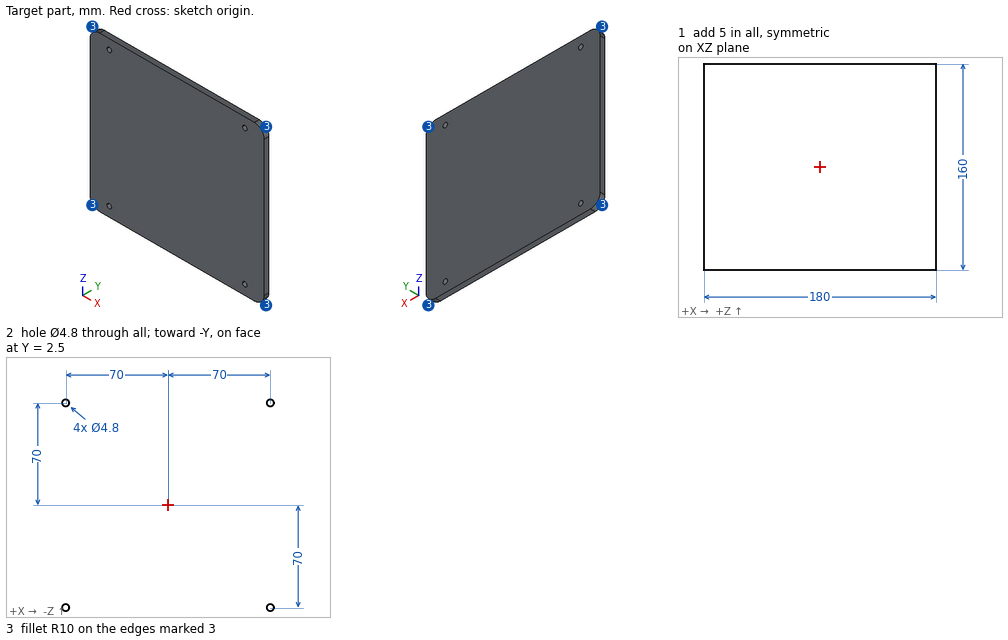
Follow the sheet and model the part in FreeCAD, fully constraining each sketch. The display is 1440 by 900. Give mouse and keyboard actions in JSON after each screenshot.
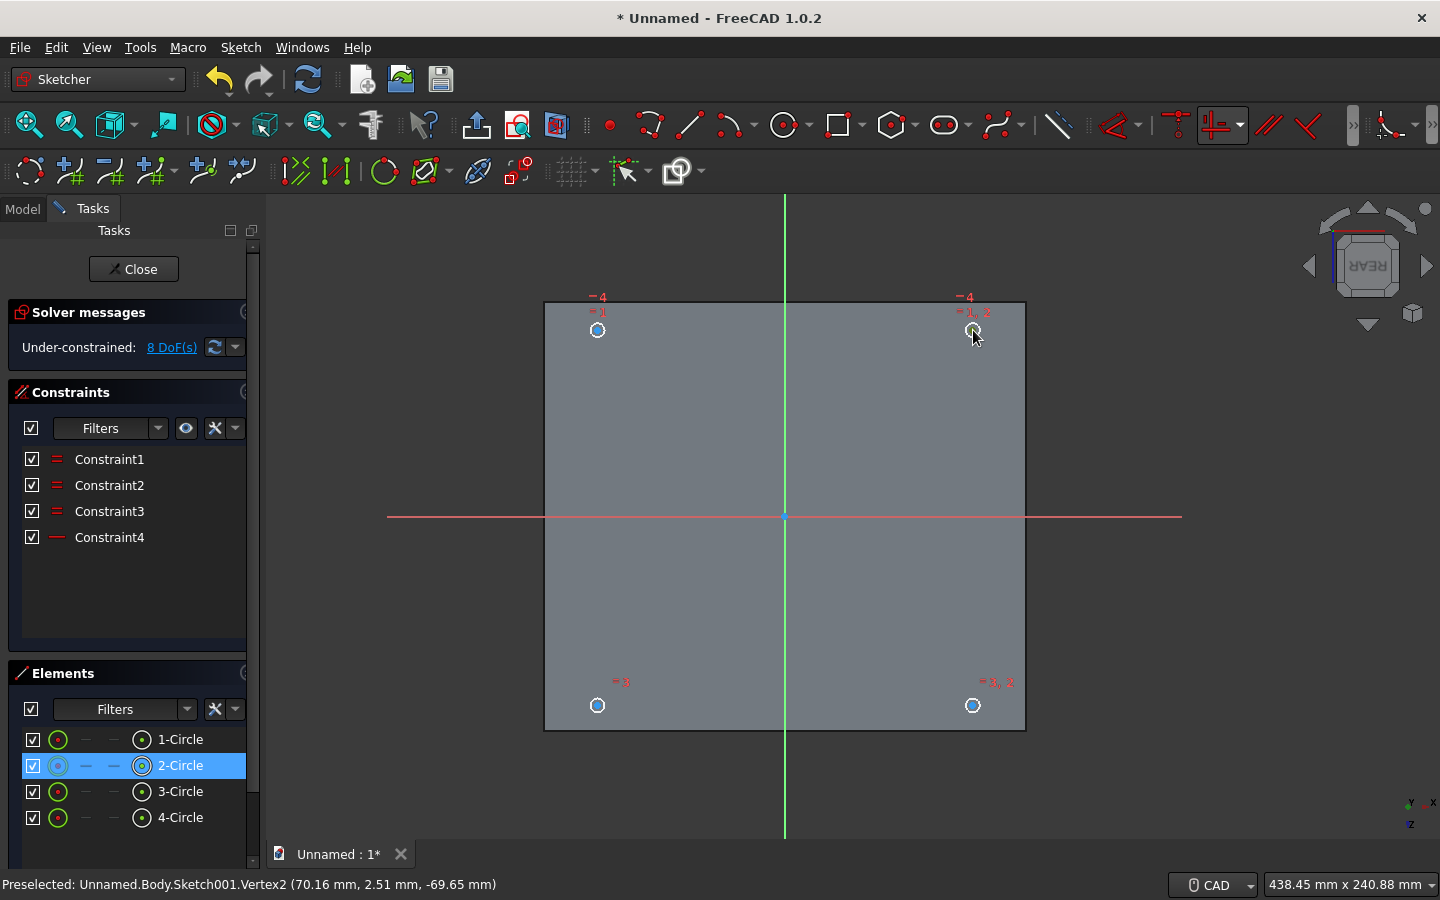
{"action": "left_click", "coordinate": [973, 705]}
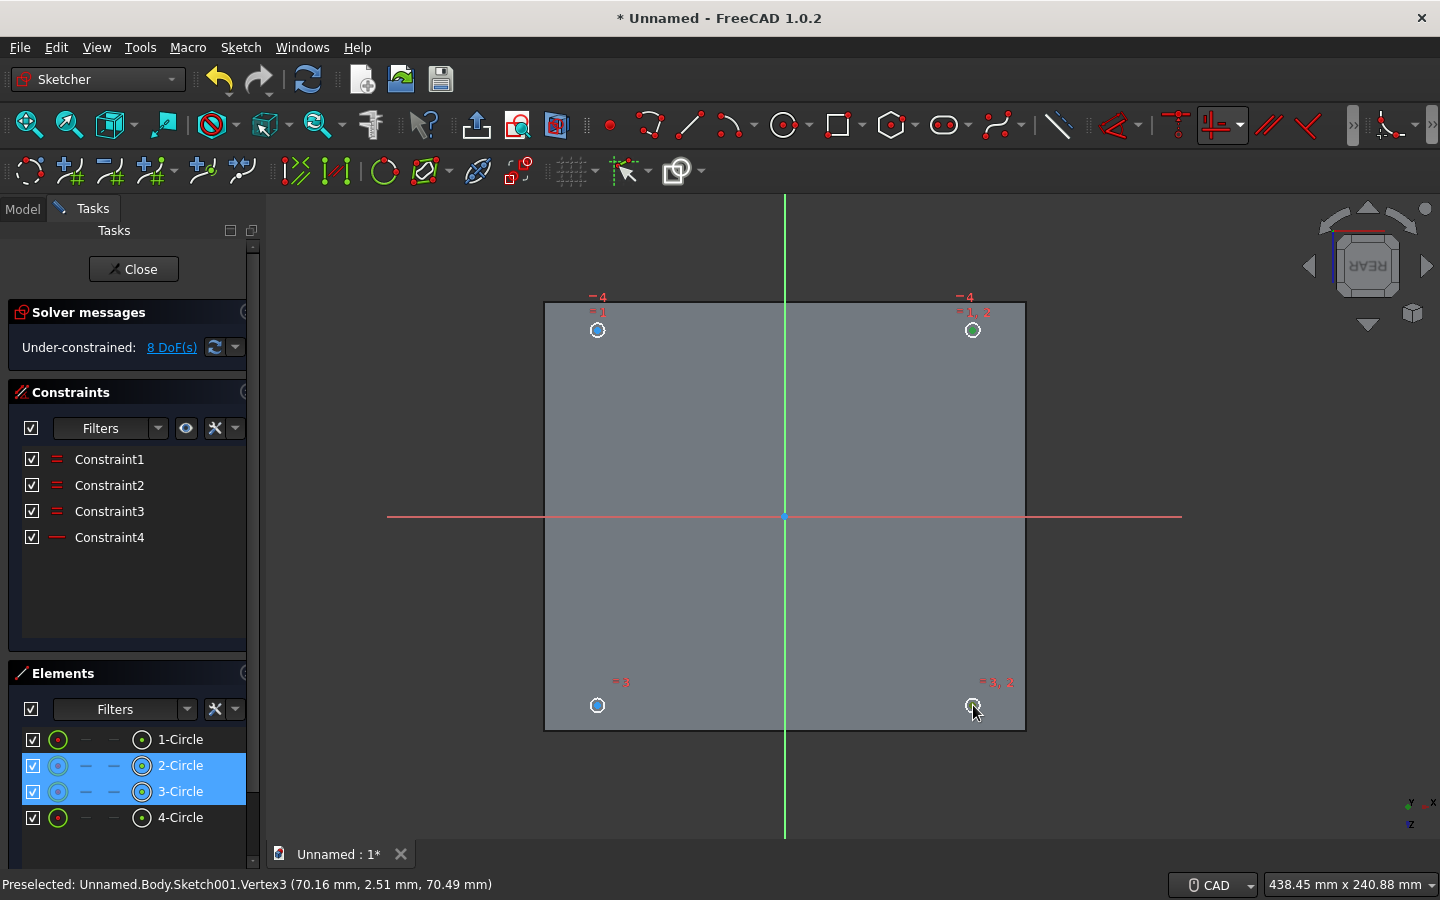
{"action": "key", "text": "v"}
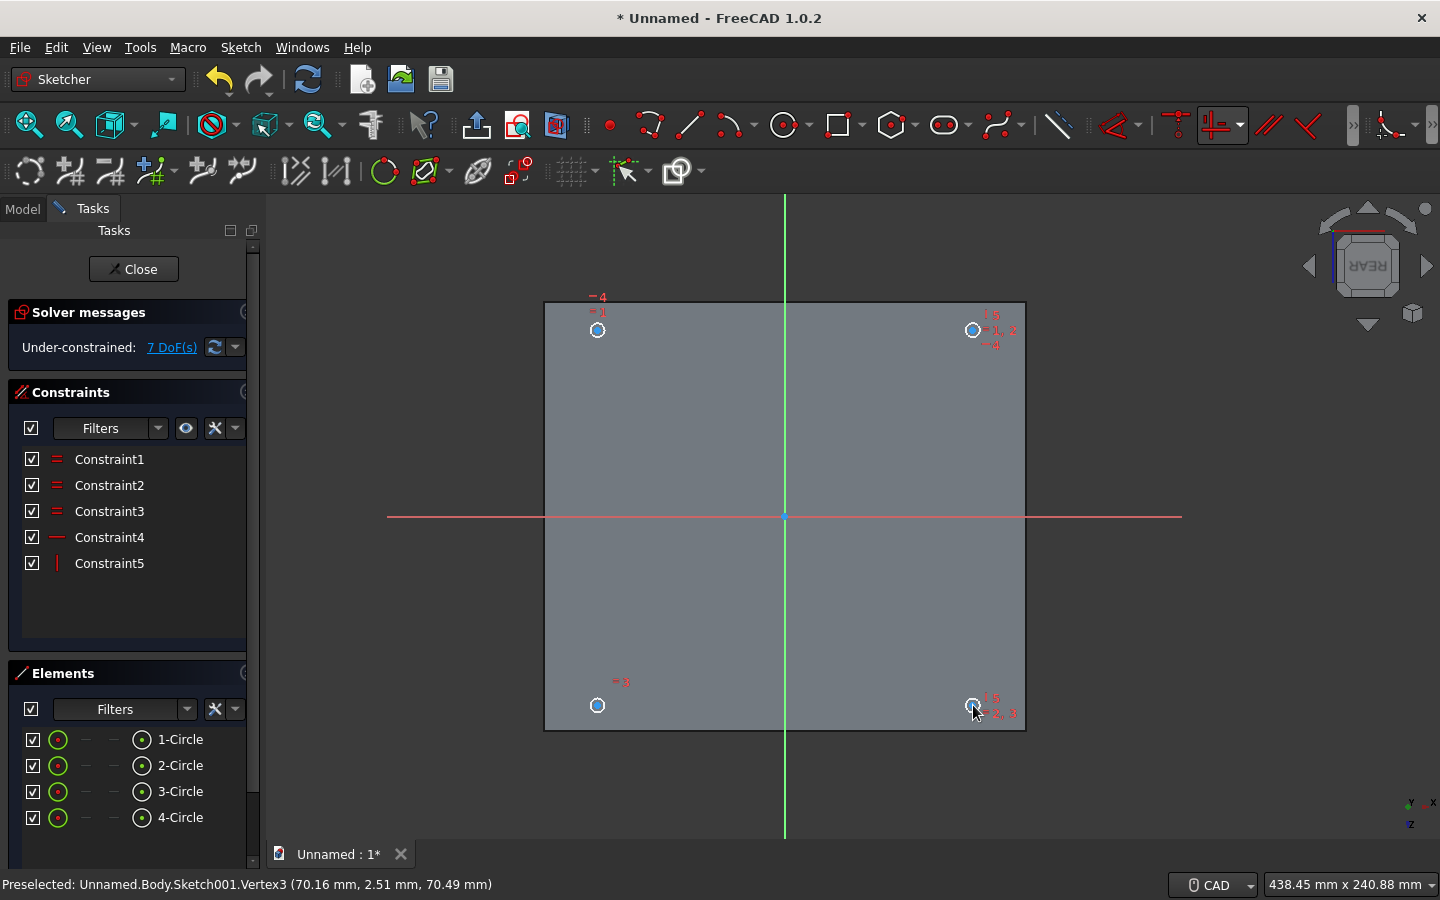
{"action": "left_click", "coordinate": [598, 330]}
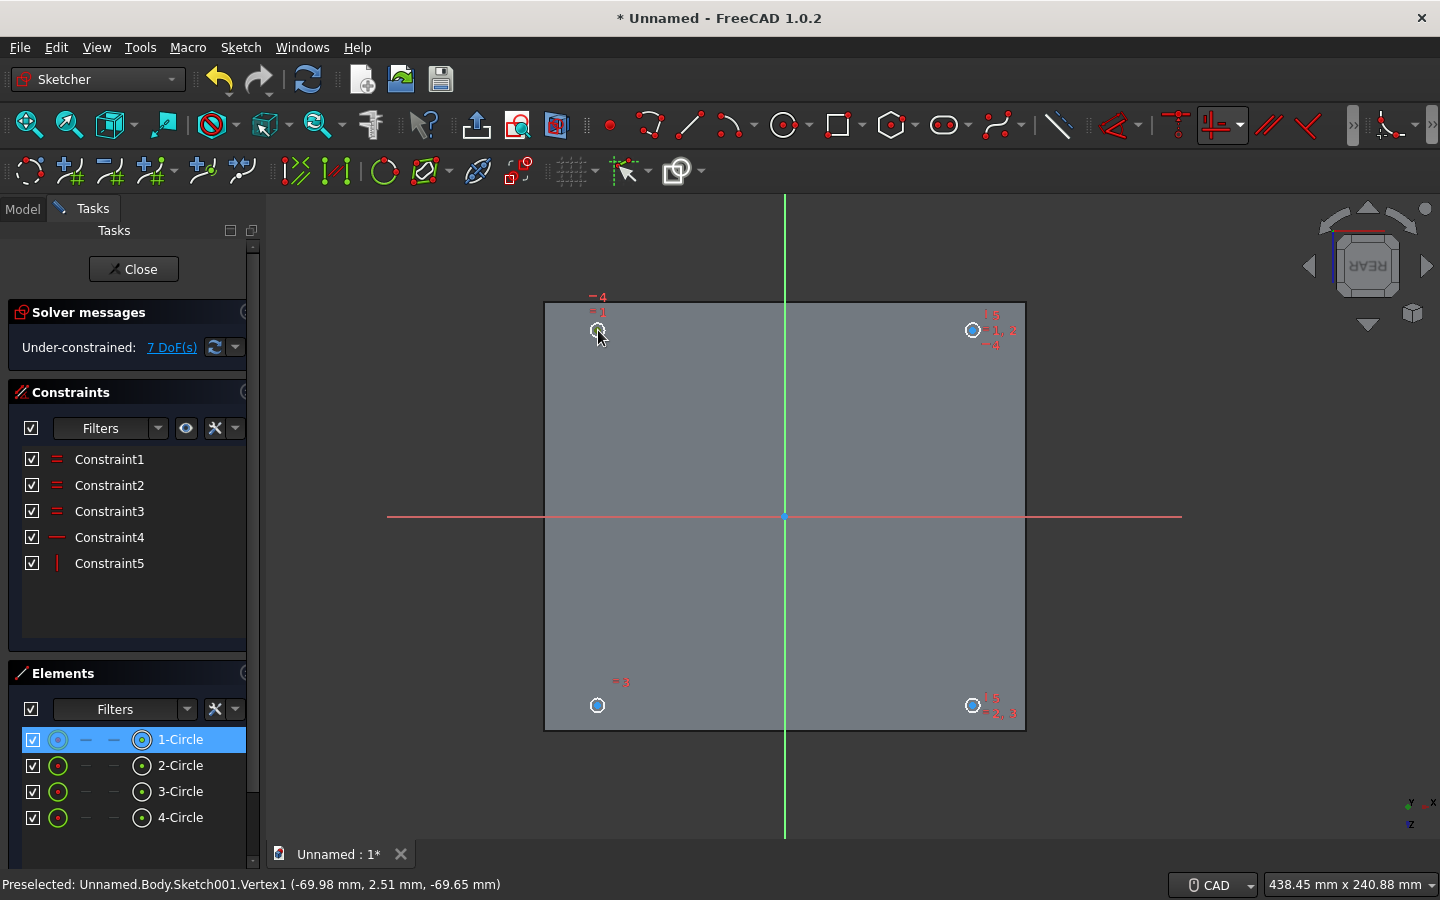
{"action": "left_click", "coordinate": [598, 705]}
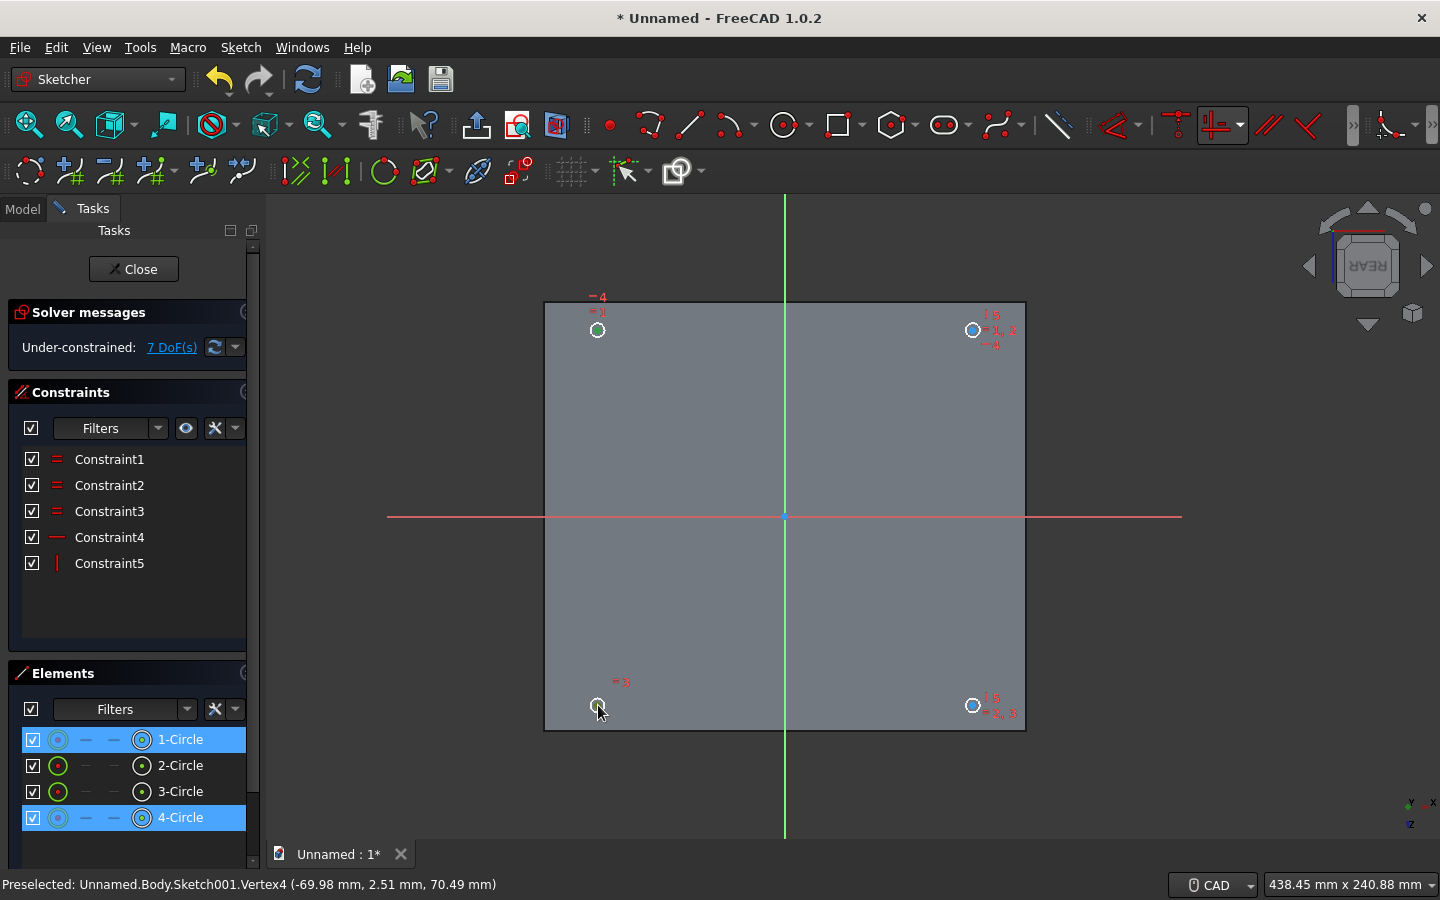
{"action": "key", "text": "v"}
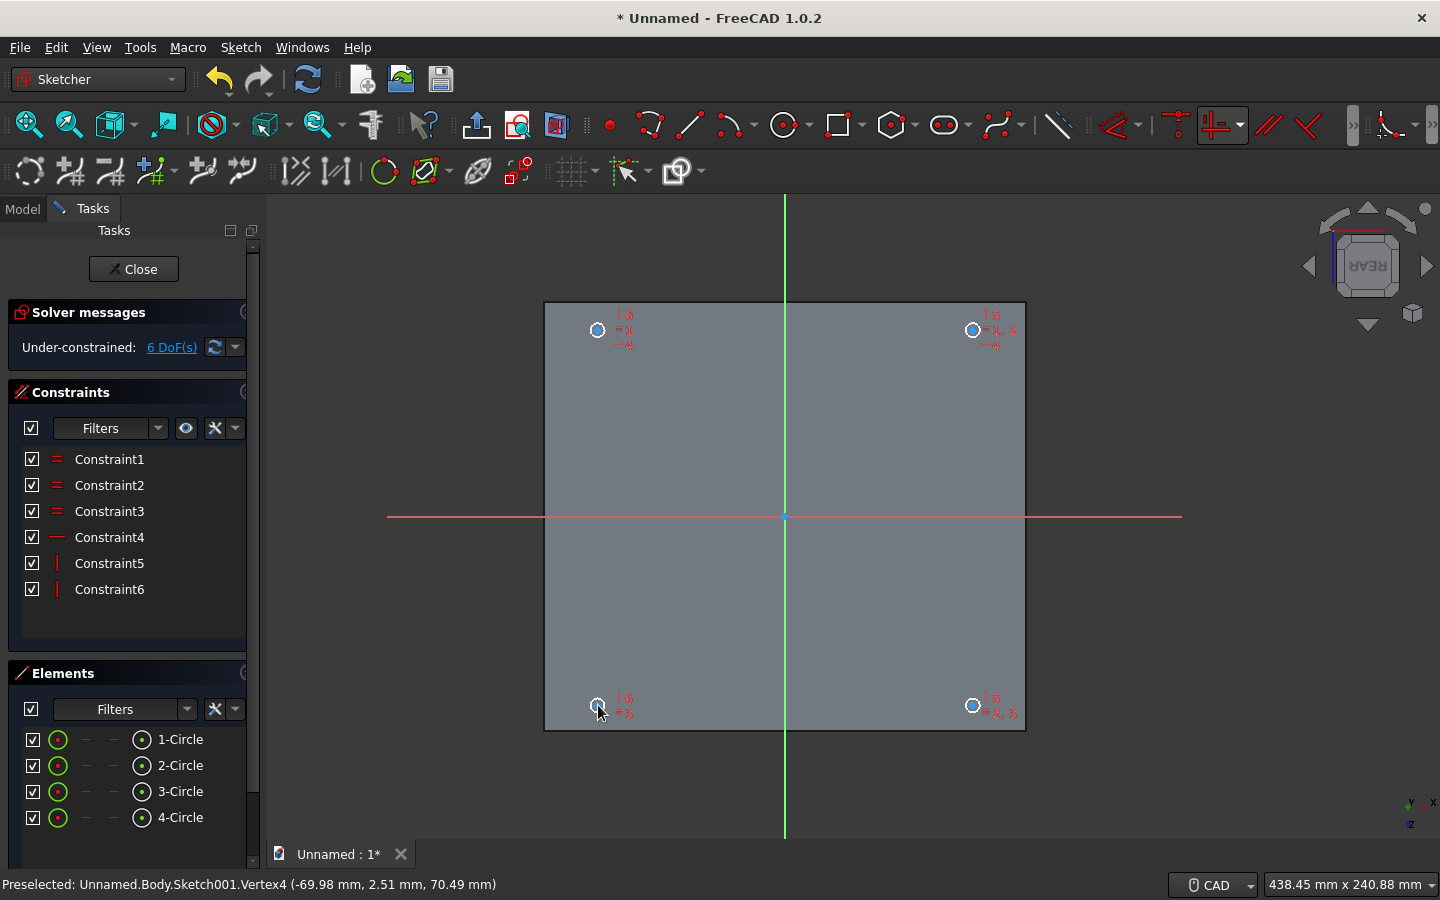
{"action": "left_click", "coordinate": [973, 705]}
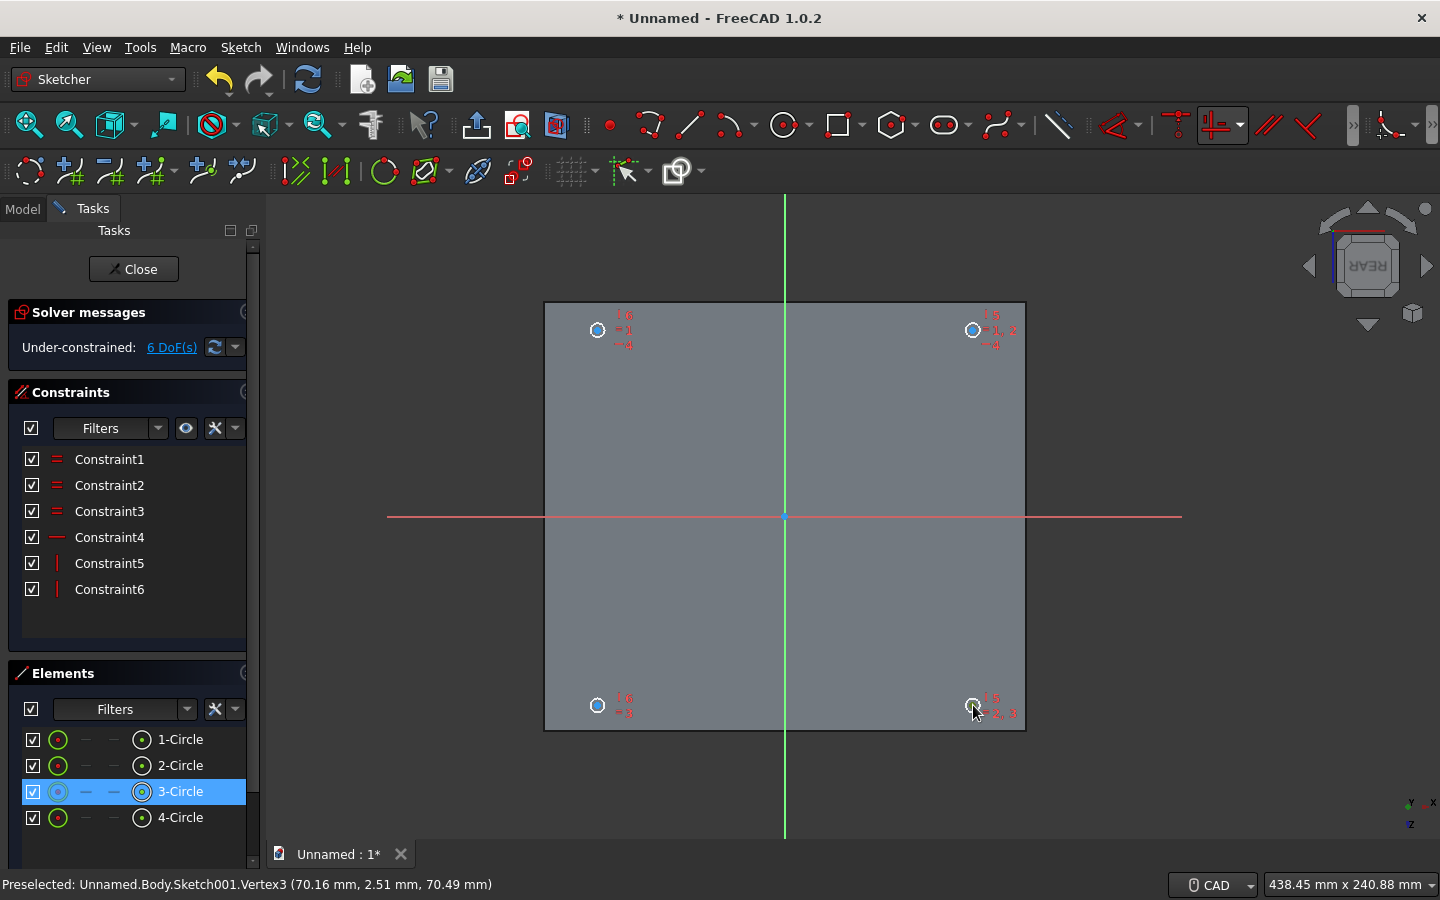
{"action": "left_click", "coordinate": [598, 705]}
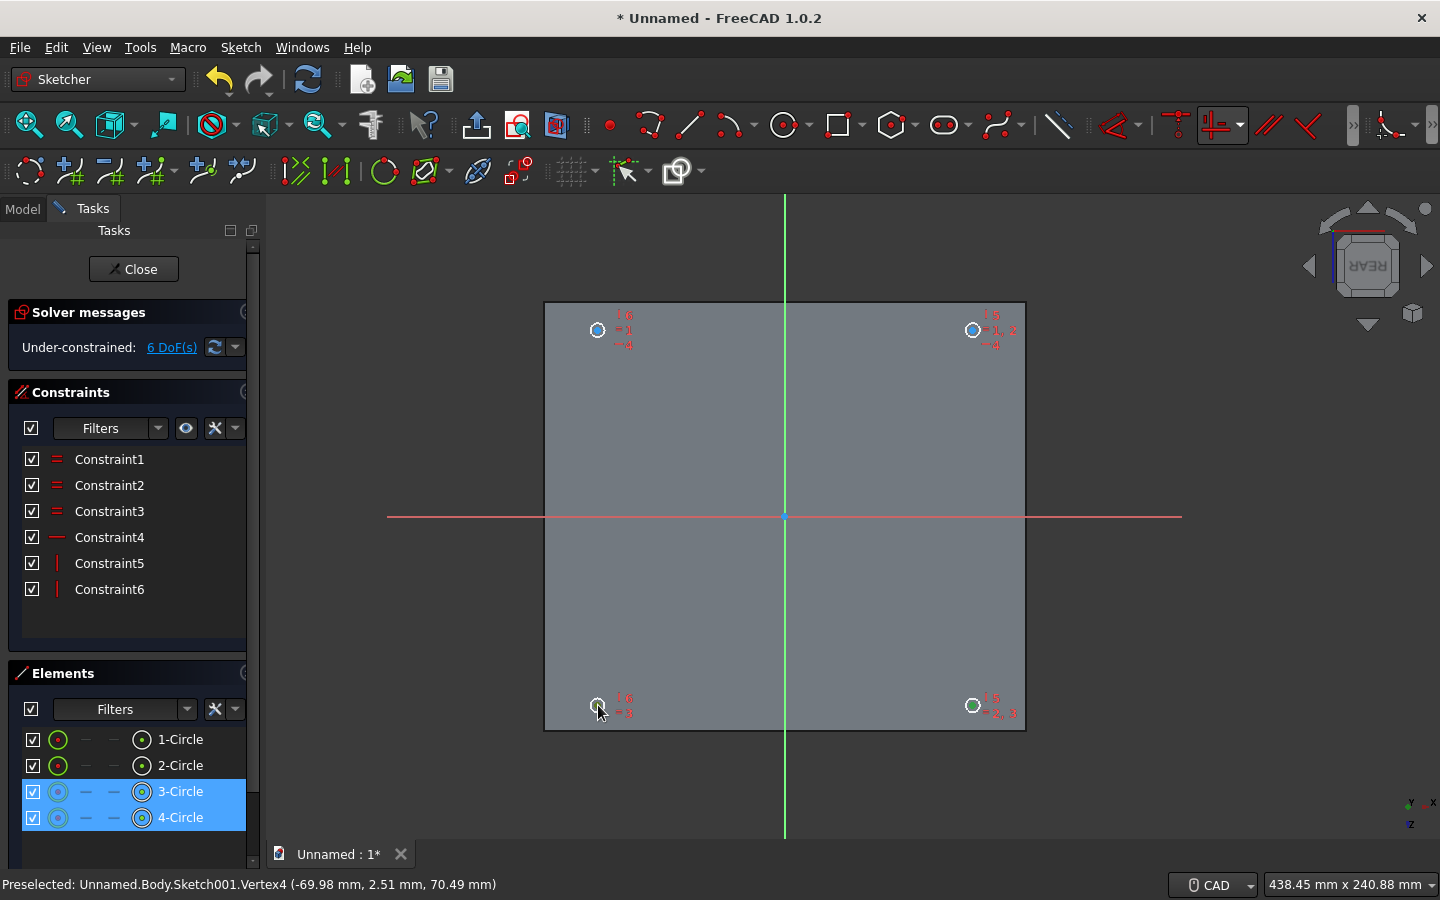
{"action": "key", "text": "h"}